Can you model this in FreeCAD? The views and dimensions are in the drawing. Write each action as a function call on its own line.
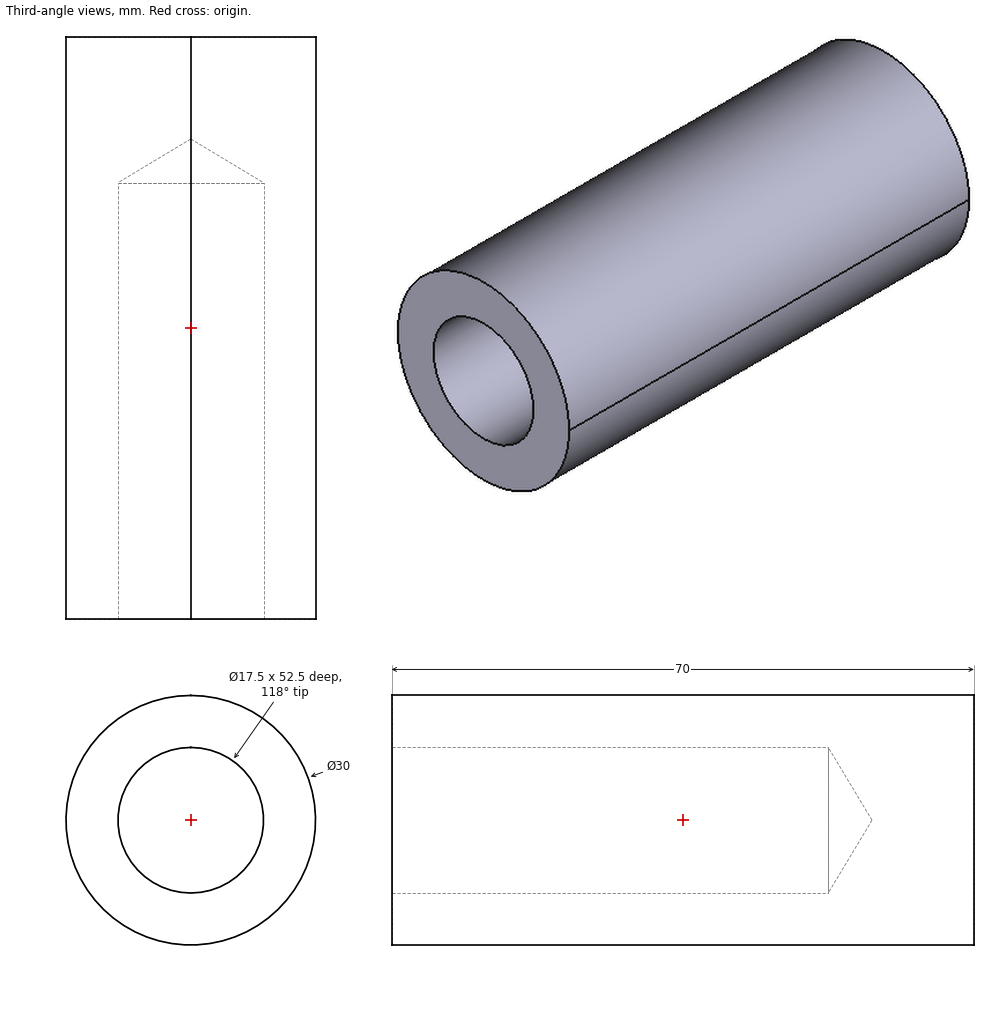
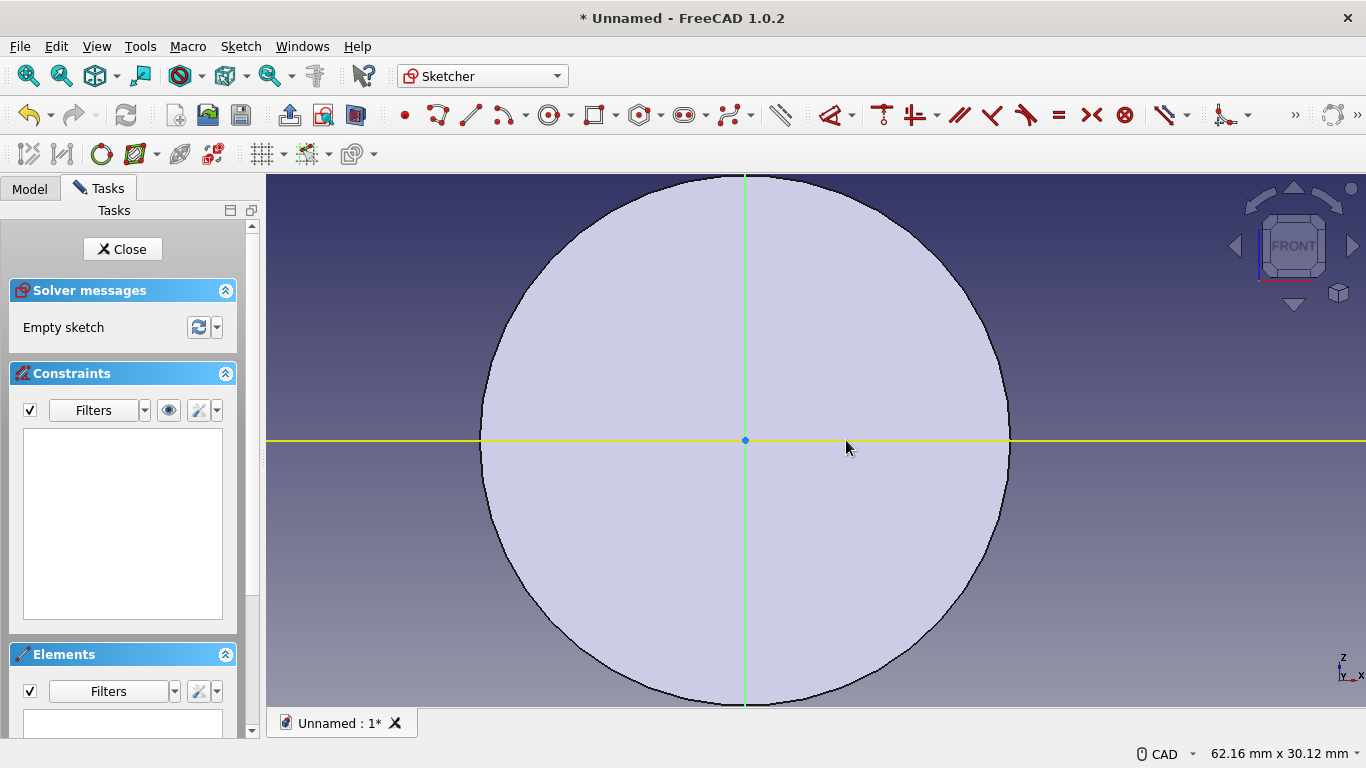
click(548, 116)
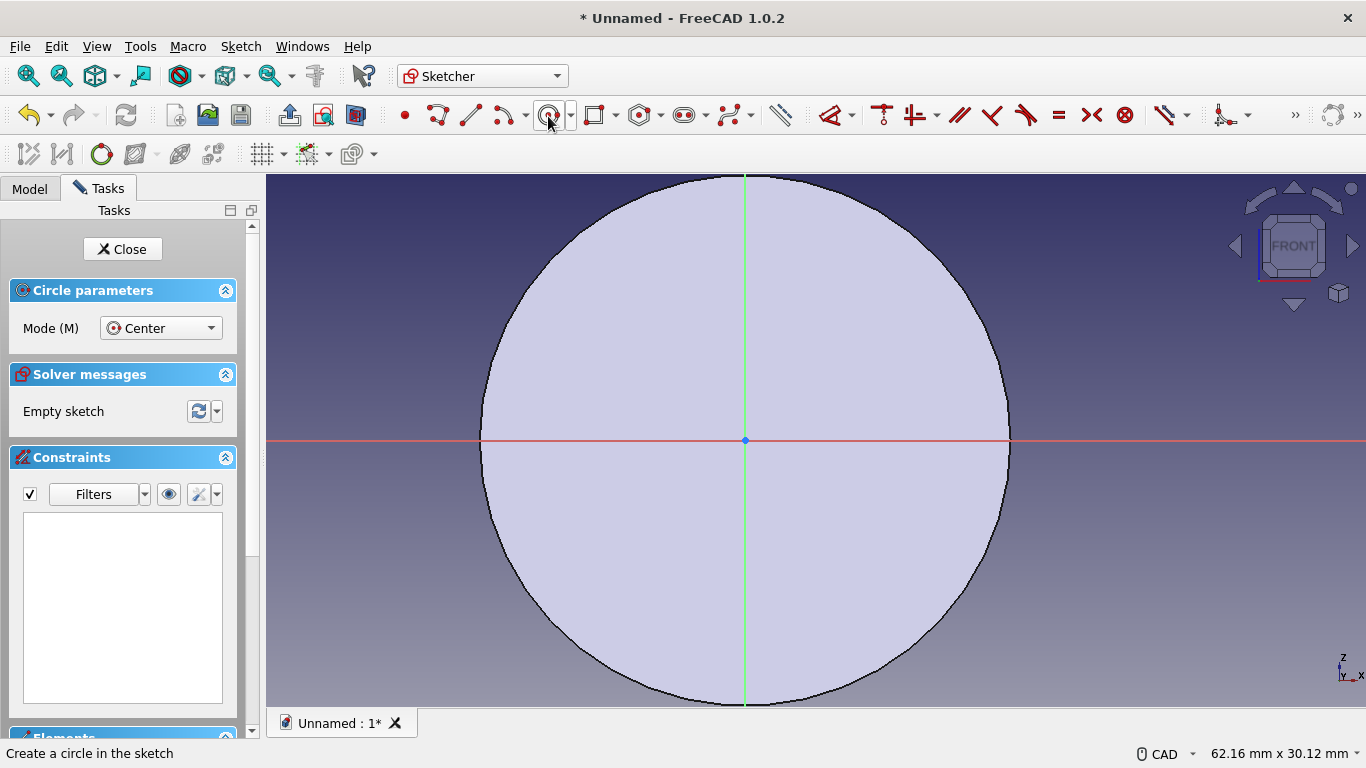
click(745, 440)
click(855, 331)
key(Escape)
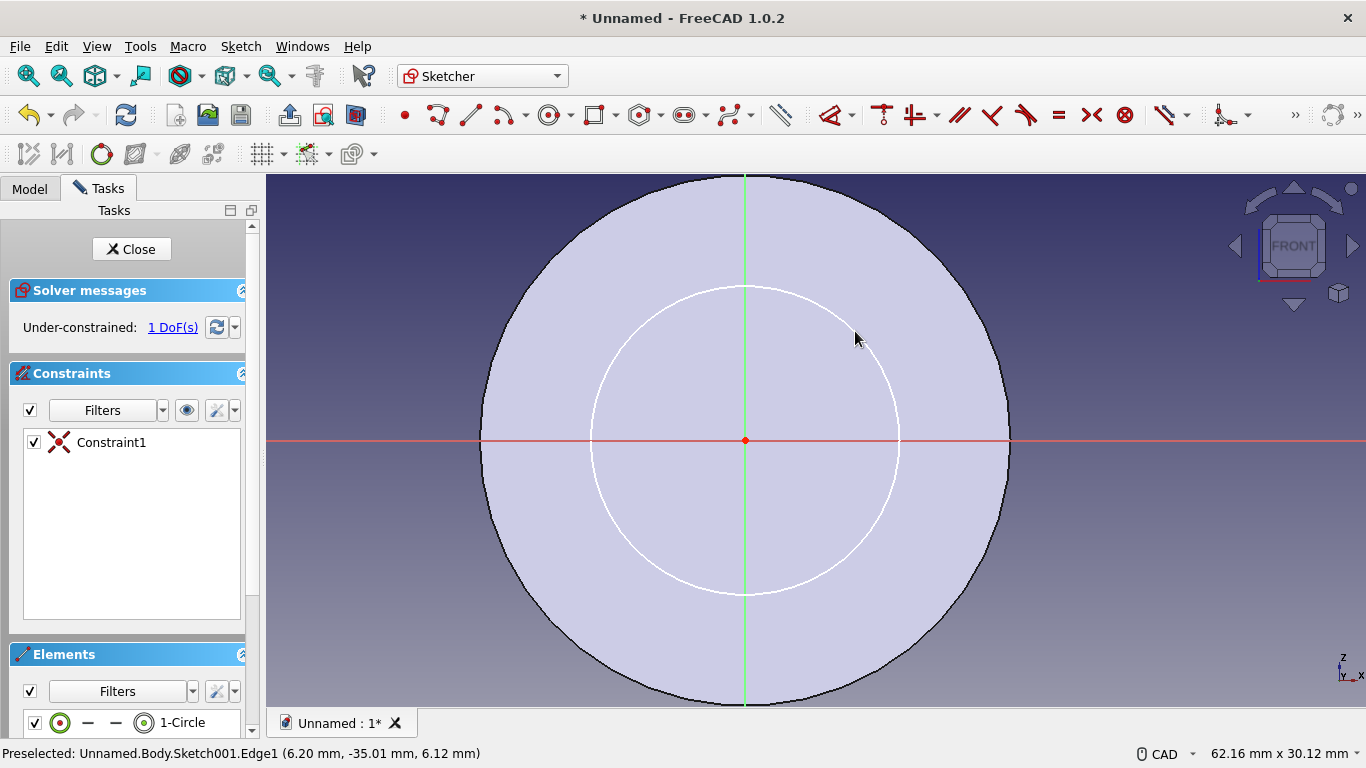
key(d)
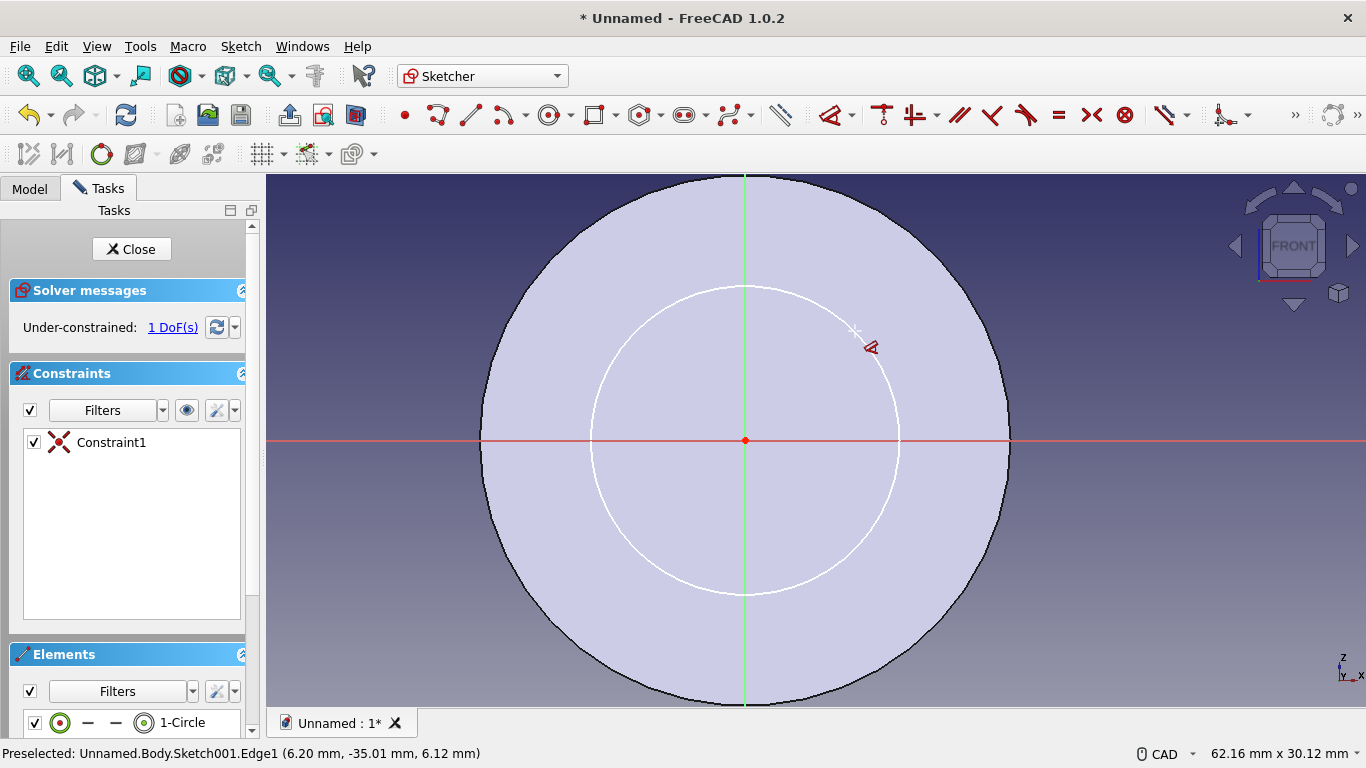
click(854, 331)
click(877, 308)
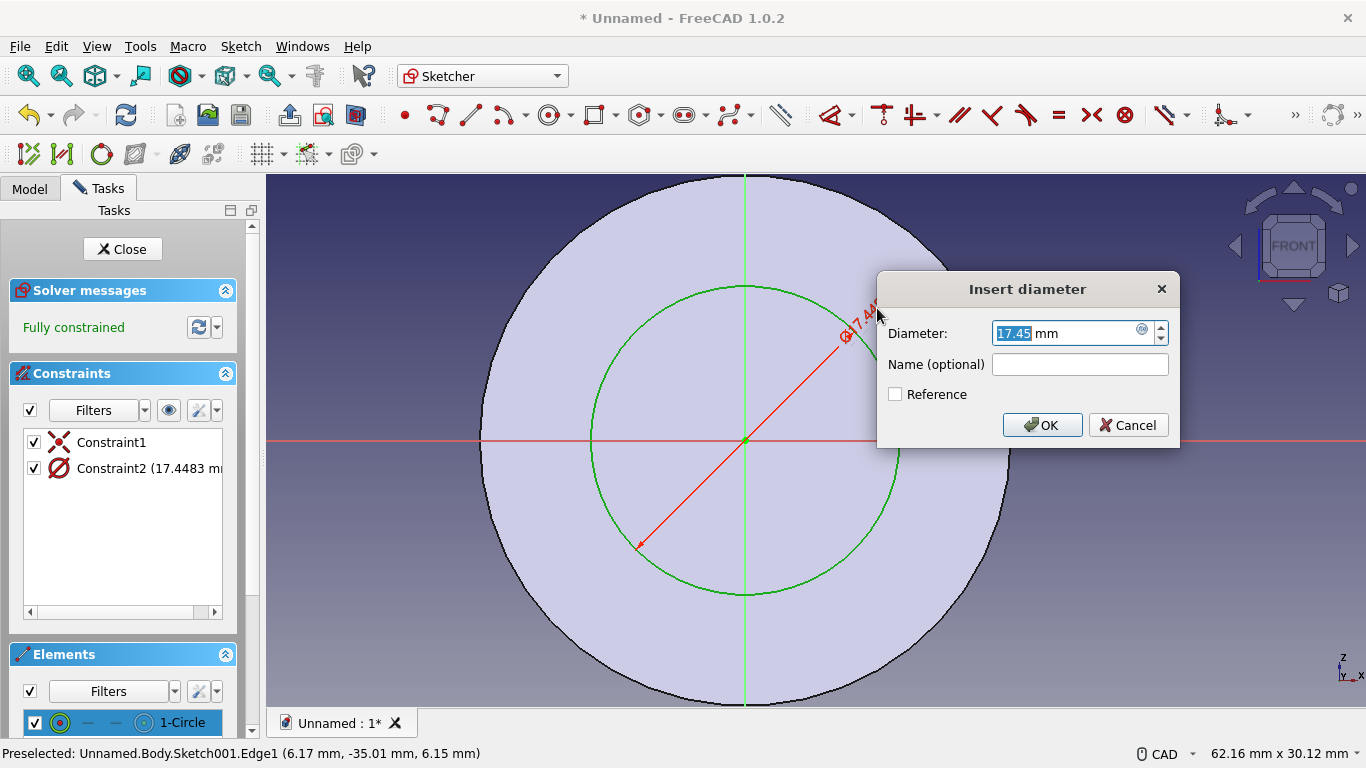
text(17.5)
key(Return)
key(Escape)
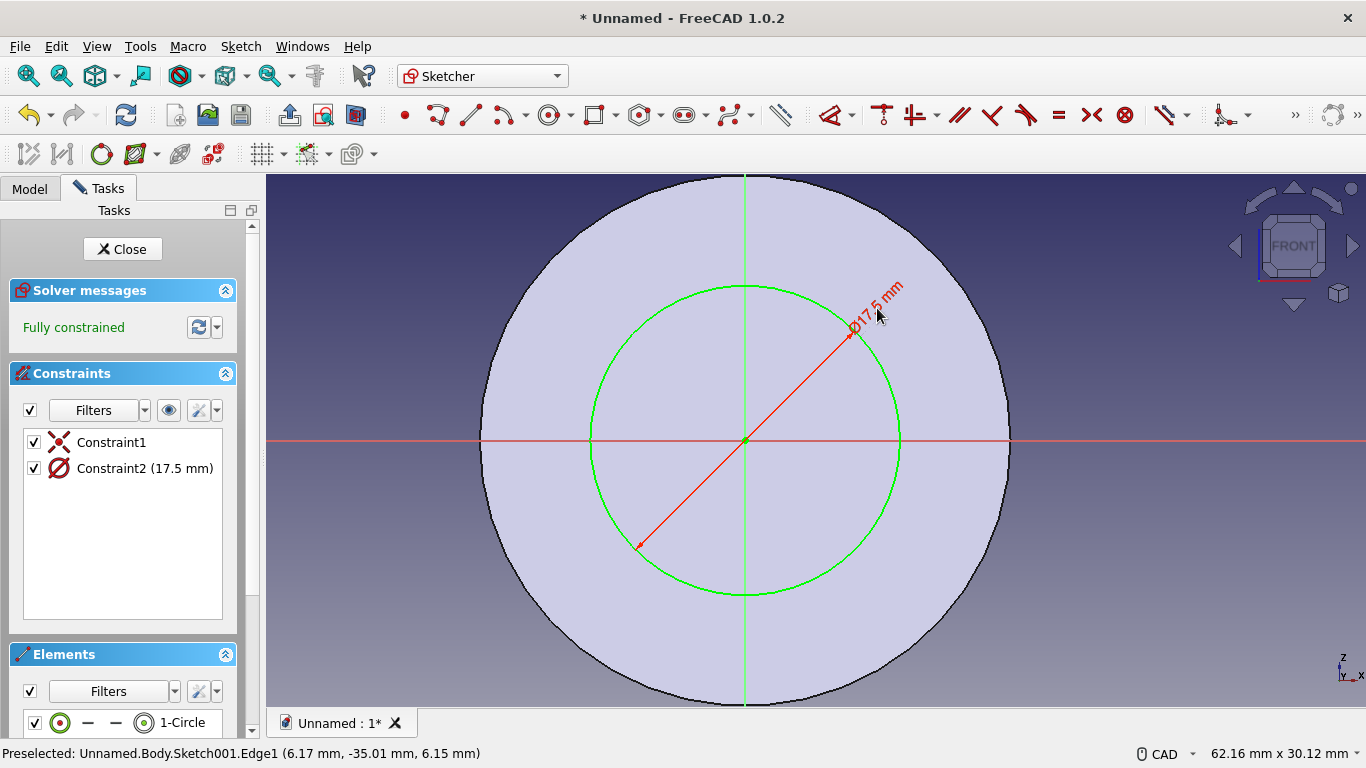
click(123, 249)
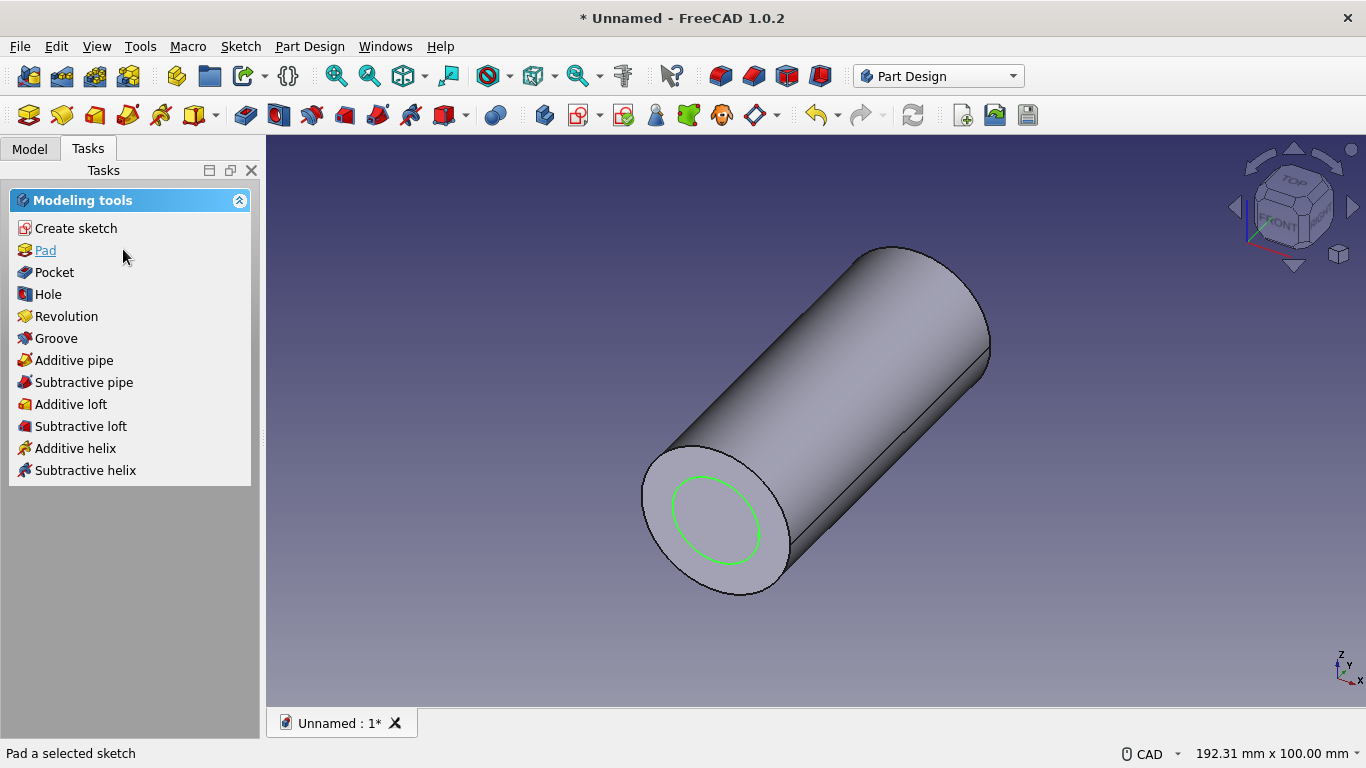
click(279, 116)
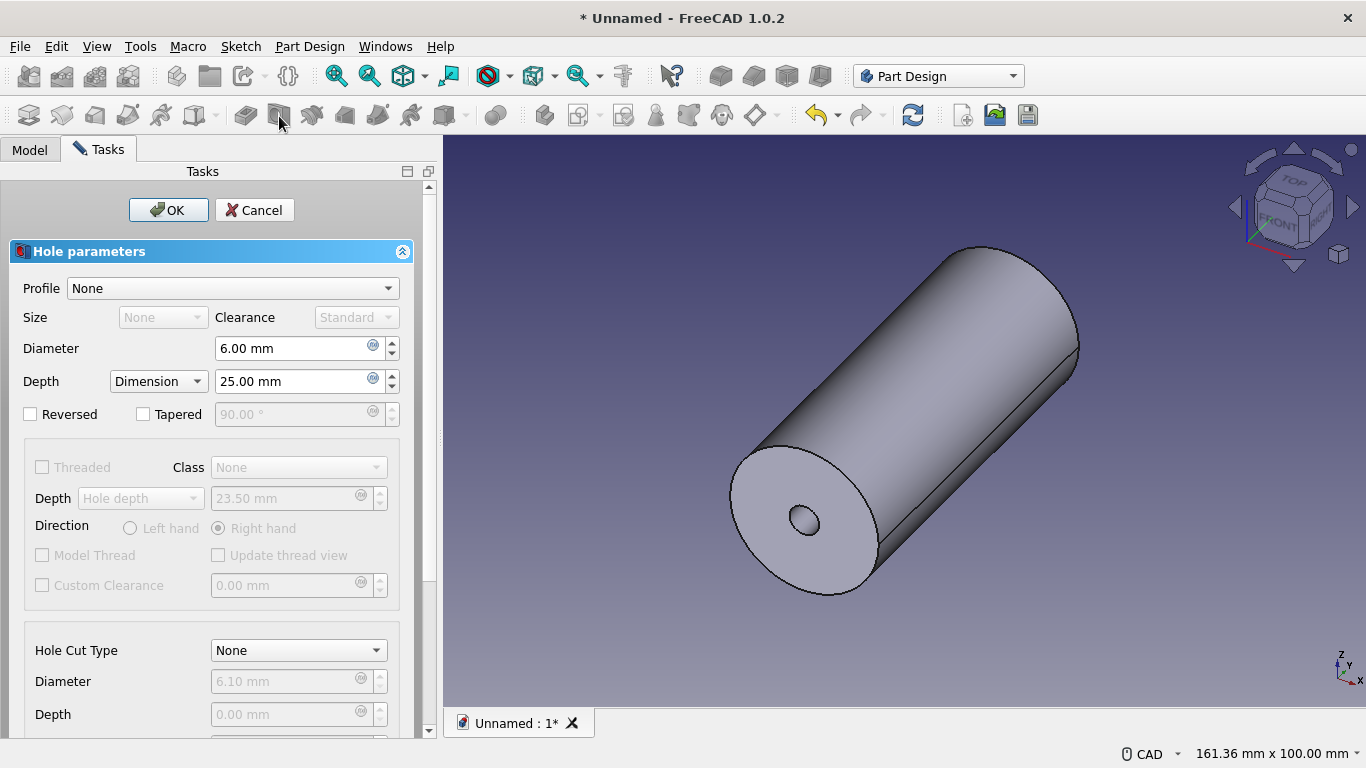
triple_click(300, 348)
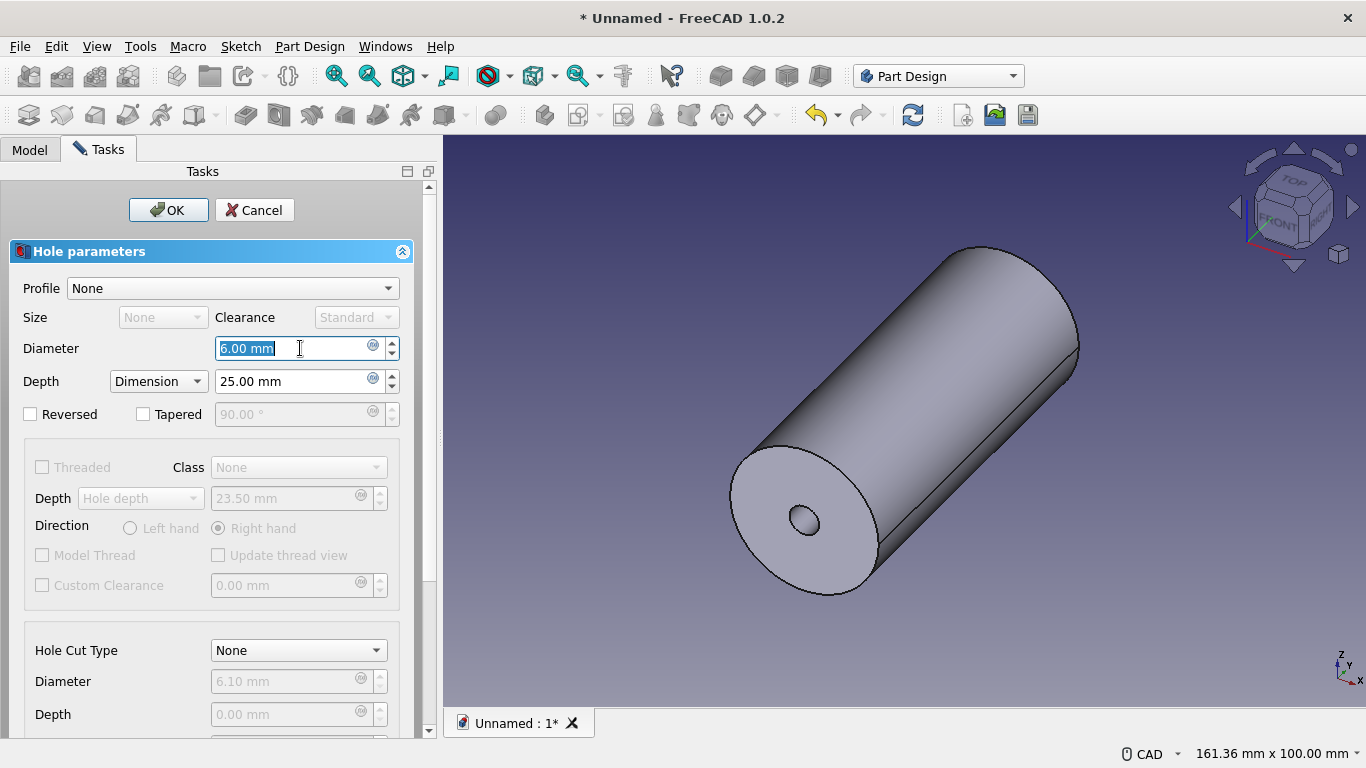
text(17.5)
key(Tab)